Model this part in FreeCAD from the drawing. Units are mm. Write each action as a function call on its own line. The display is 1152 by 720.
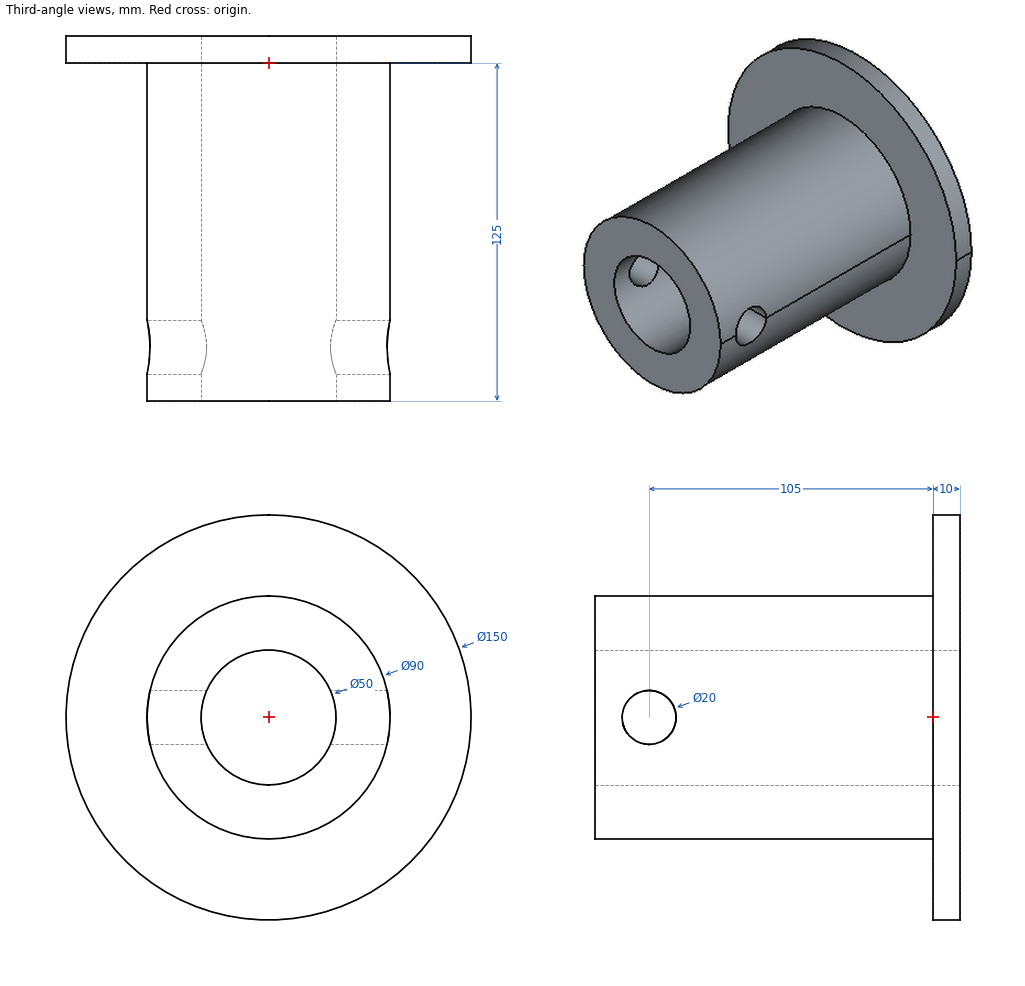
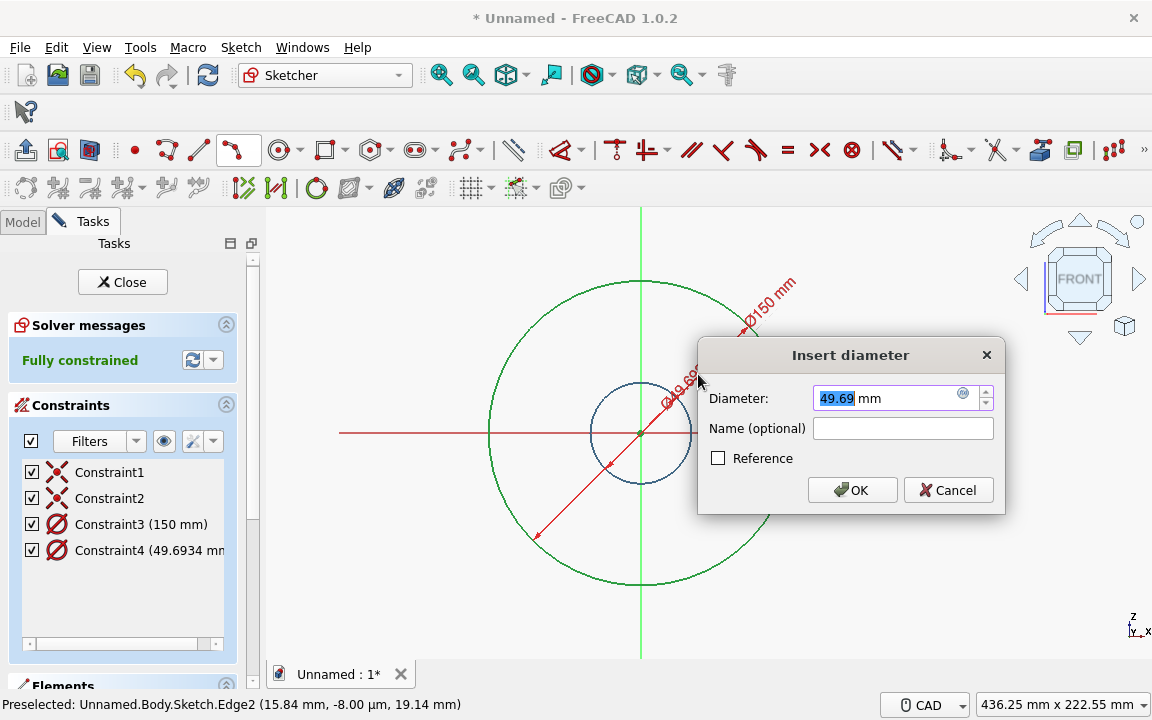
text(50)
key(Return)
key(Escape)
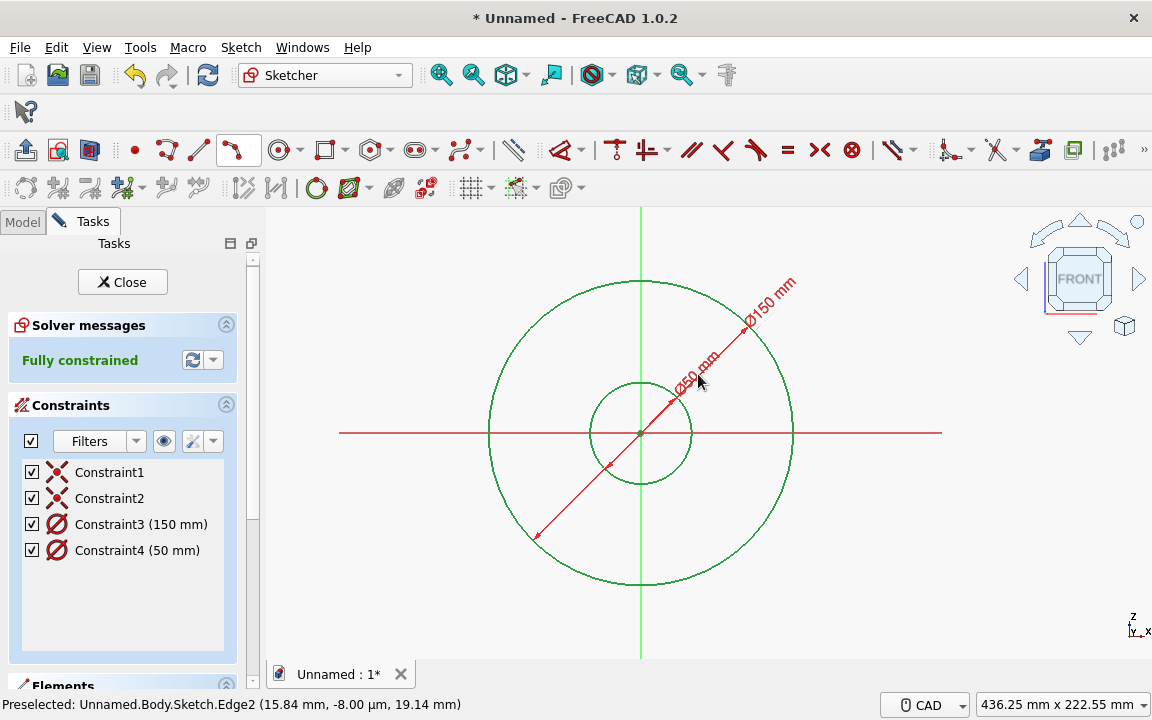
click(123, 282)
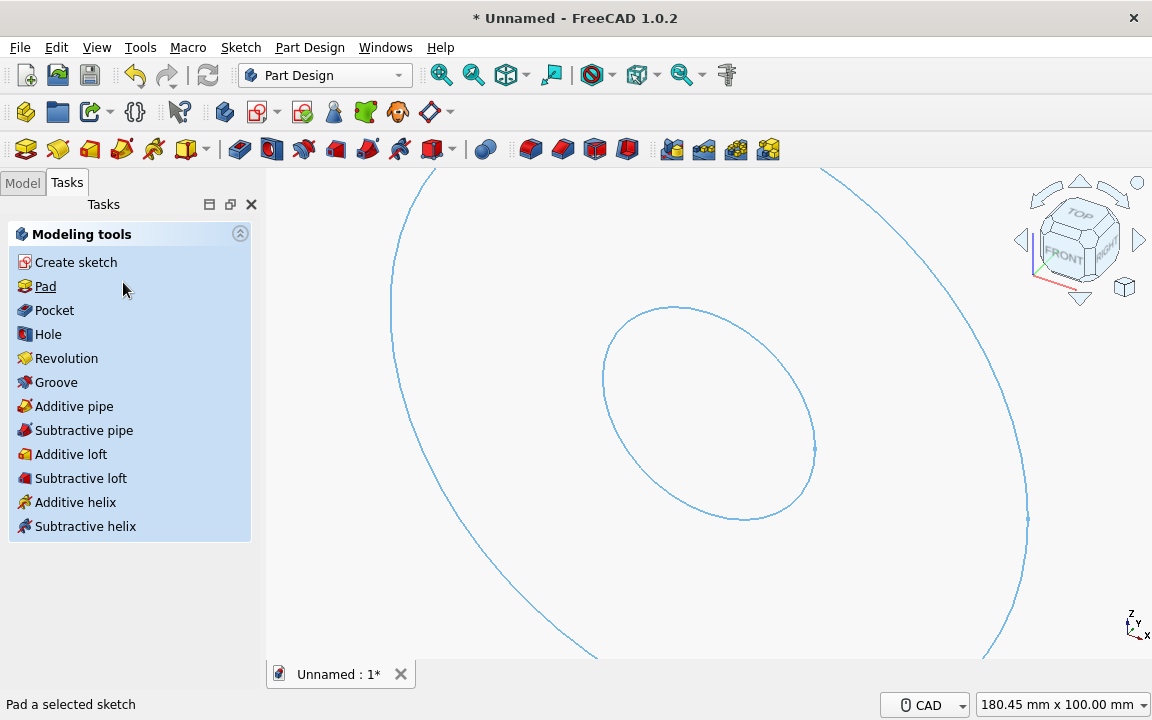
click(26, 150)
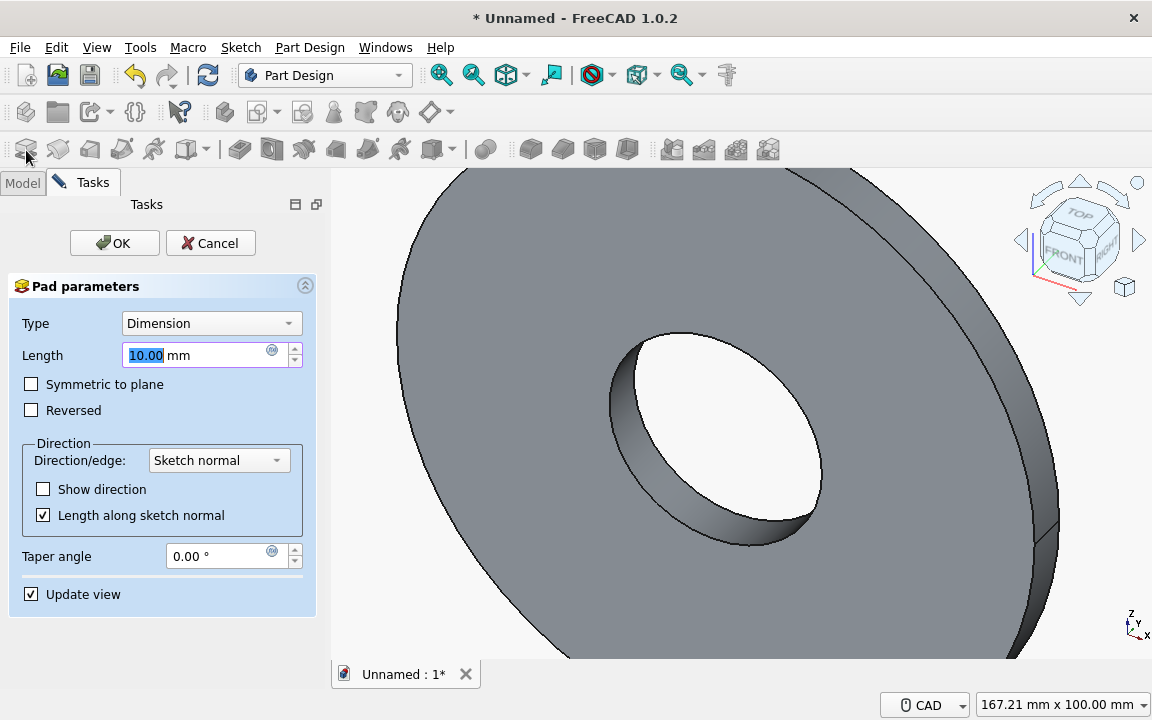
text(10)
key(Tab)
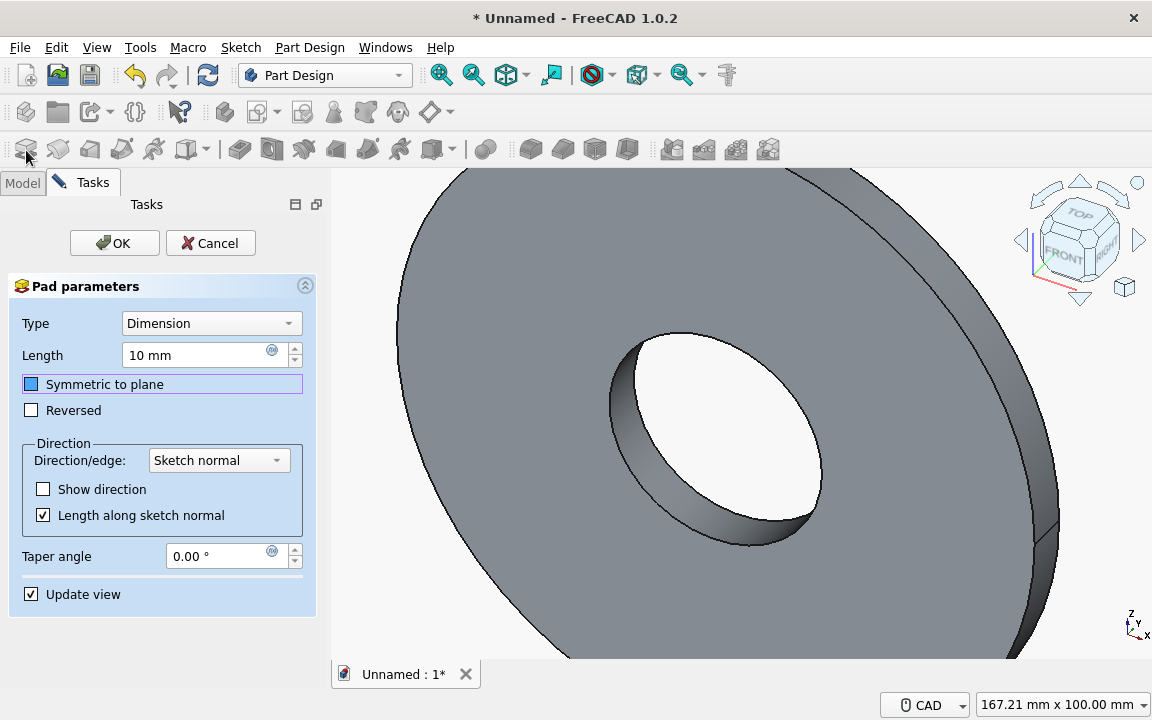
click(30, 410)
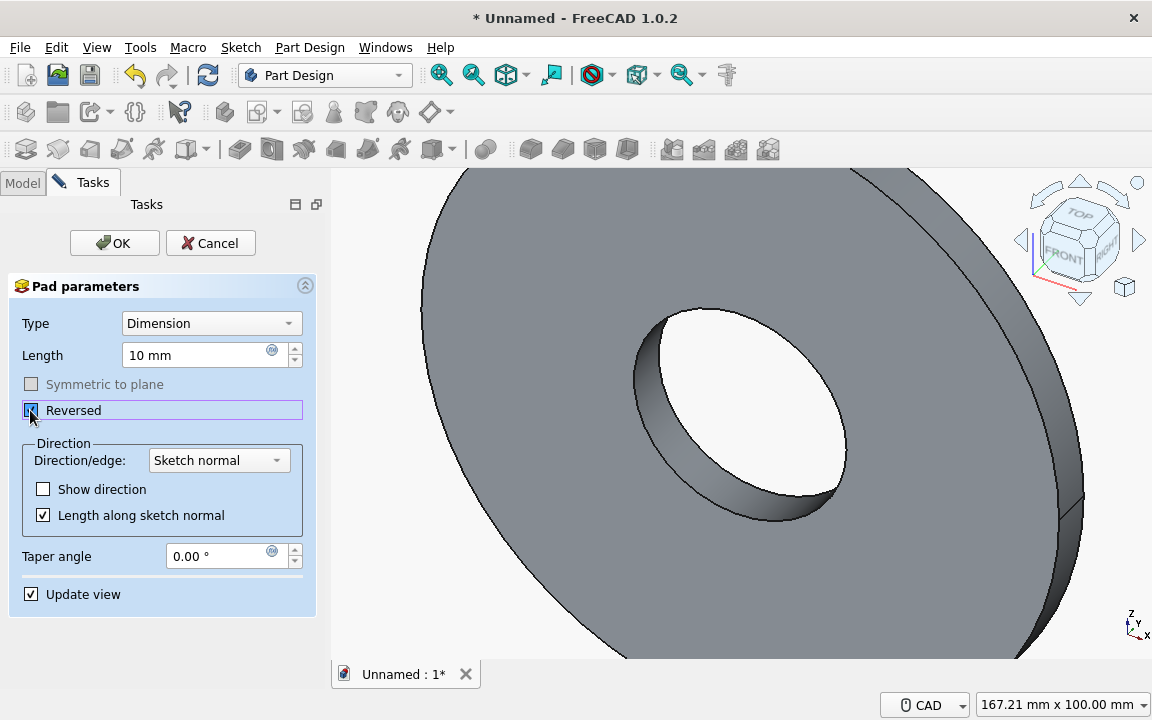
click(115, 243)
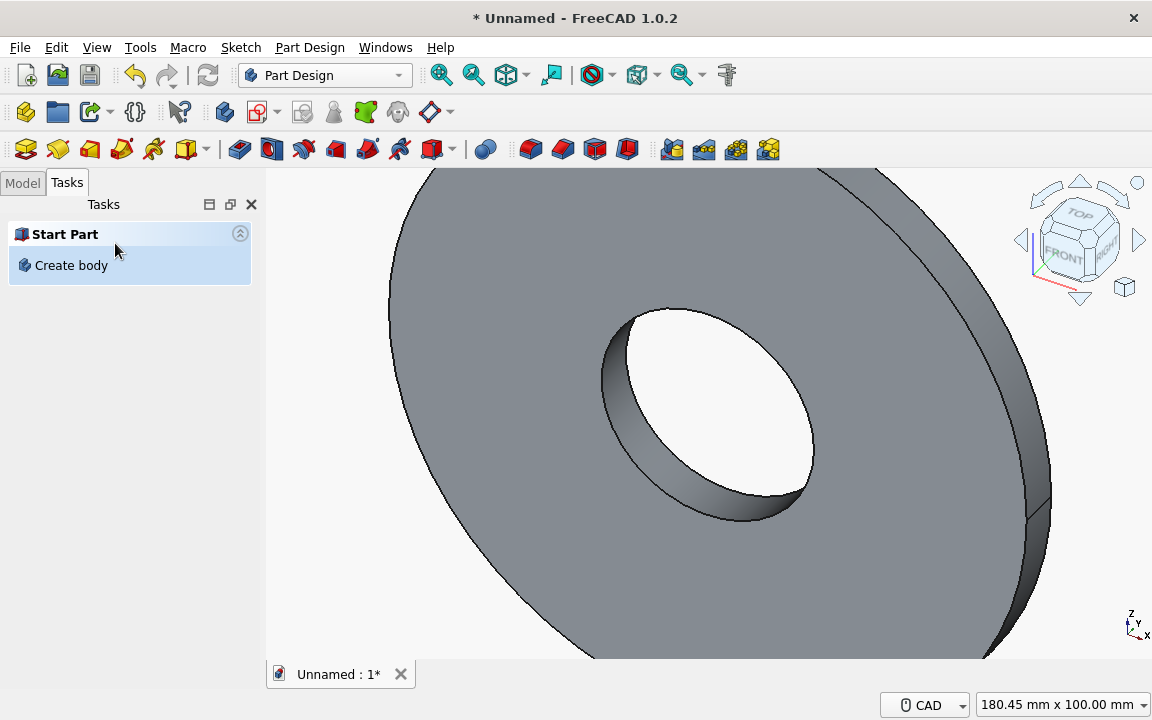
click(442, 76)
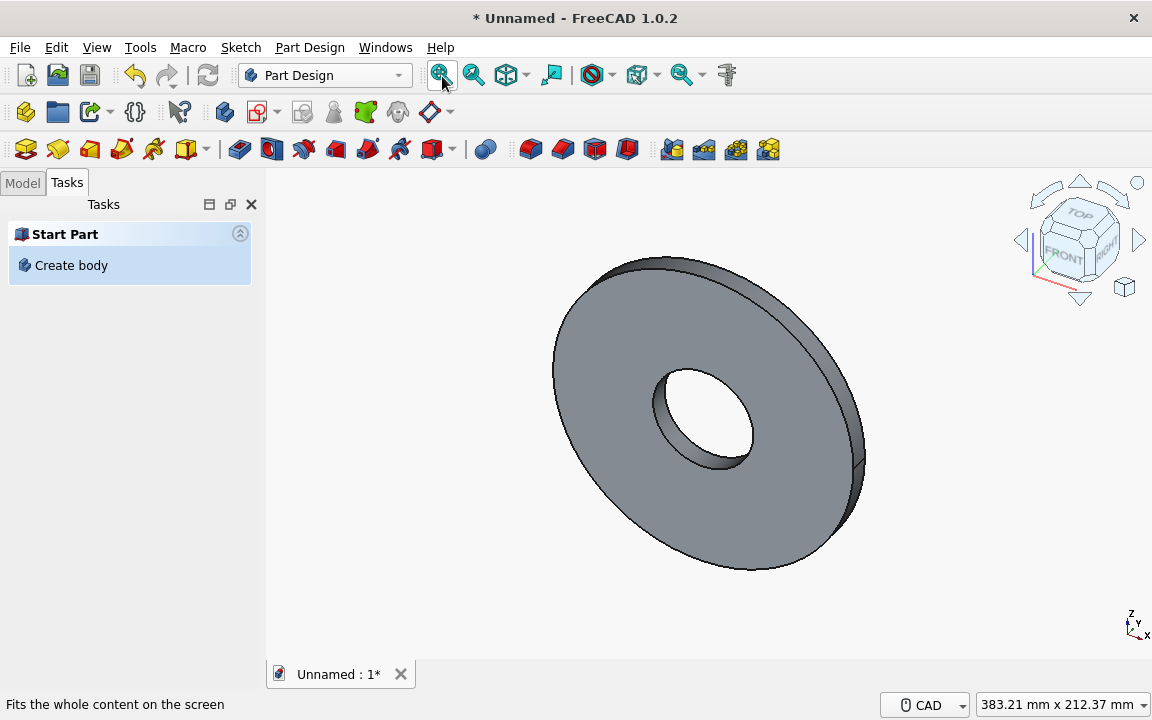
click(23, 182)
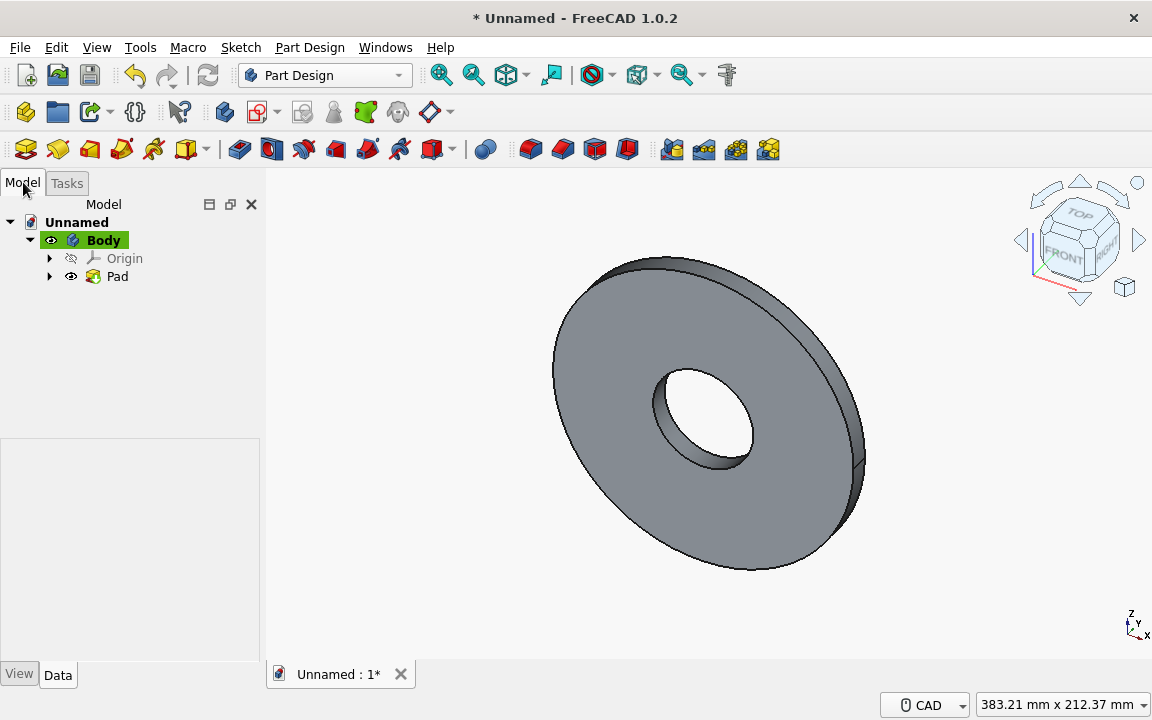
click(50, 258)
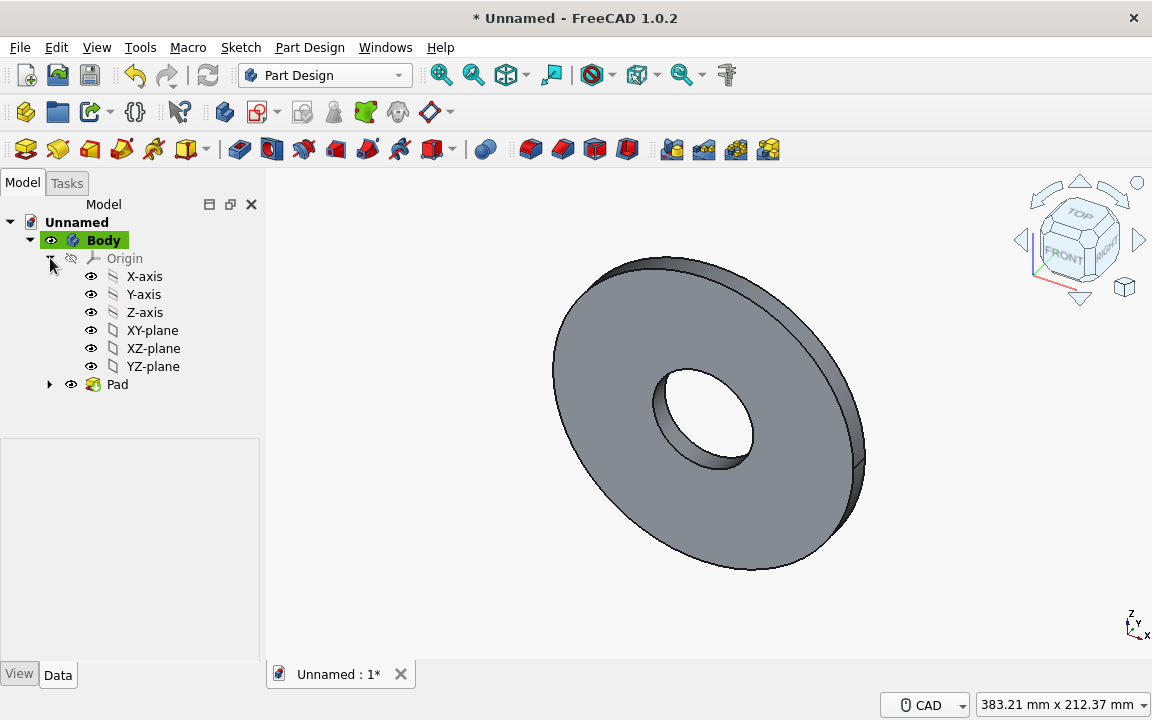
click(136, 348)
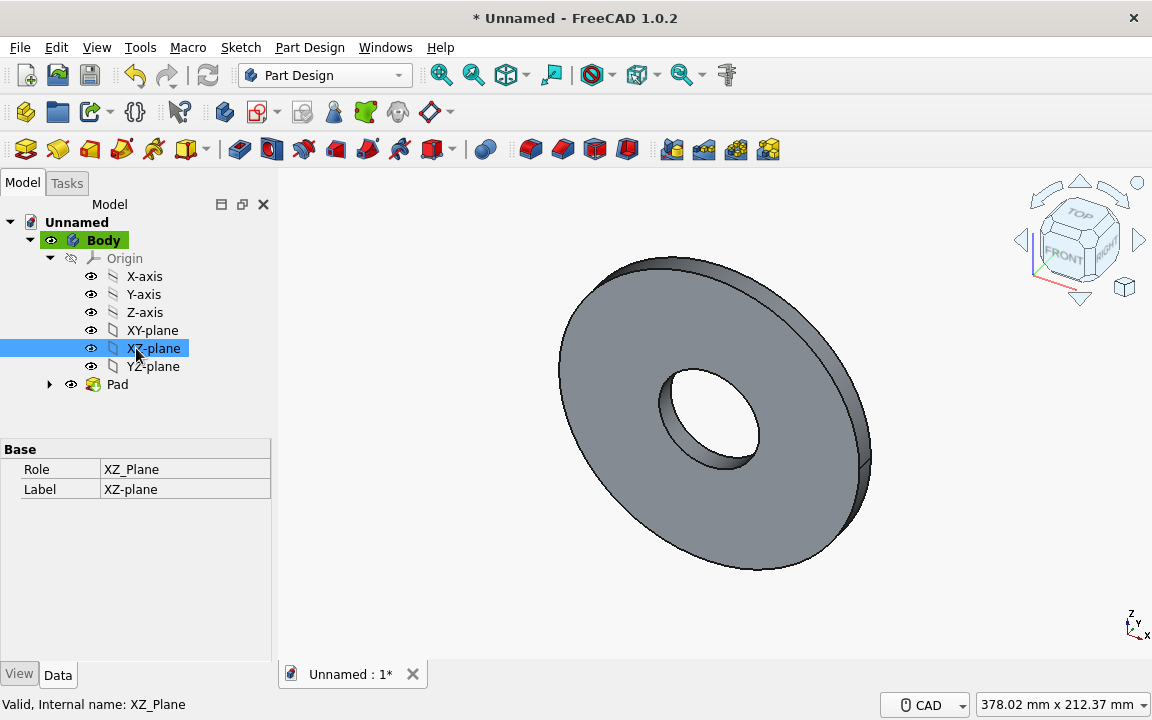
click(430, 112)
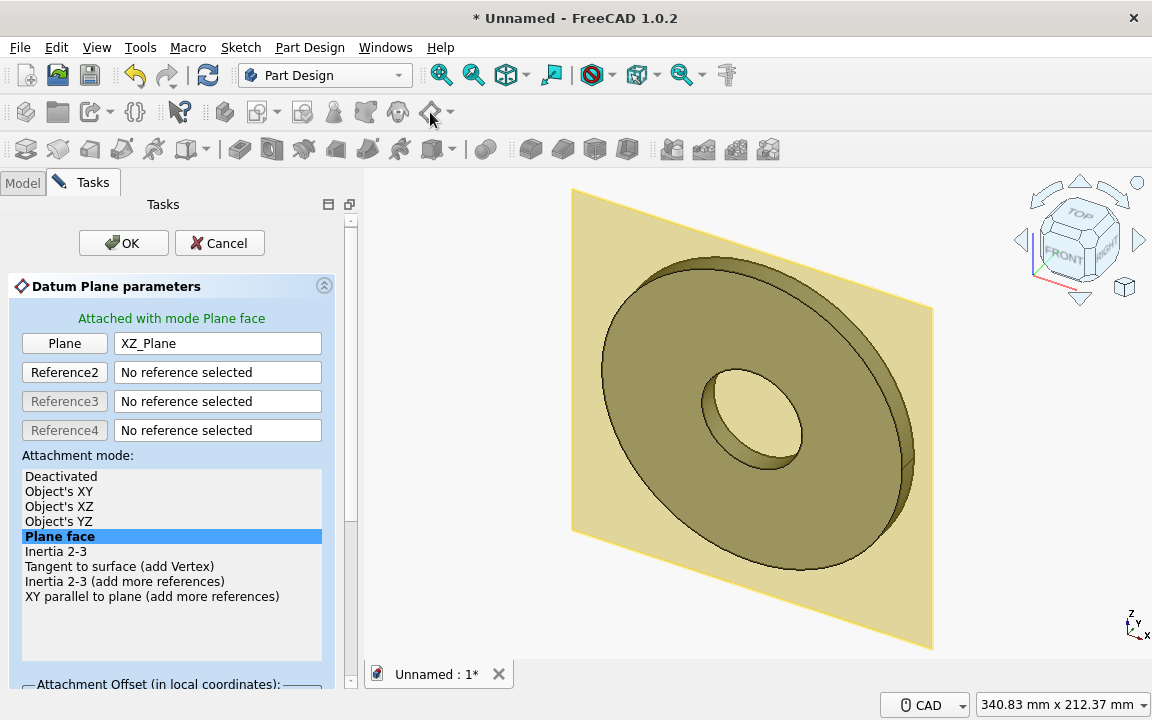
scroll(351, 451, down, 3)